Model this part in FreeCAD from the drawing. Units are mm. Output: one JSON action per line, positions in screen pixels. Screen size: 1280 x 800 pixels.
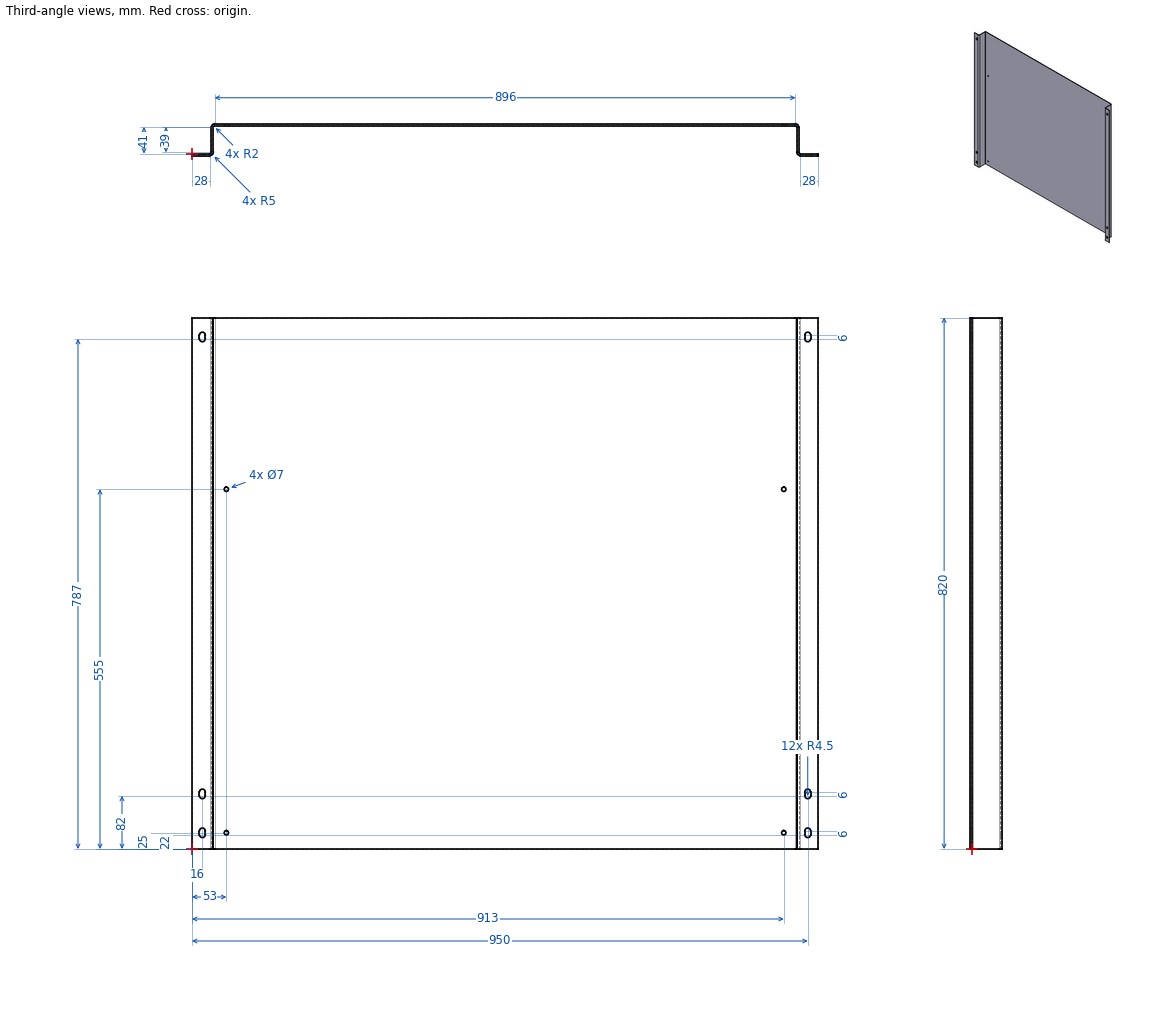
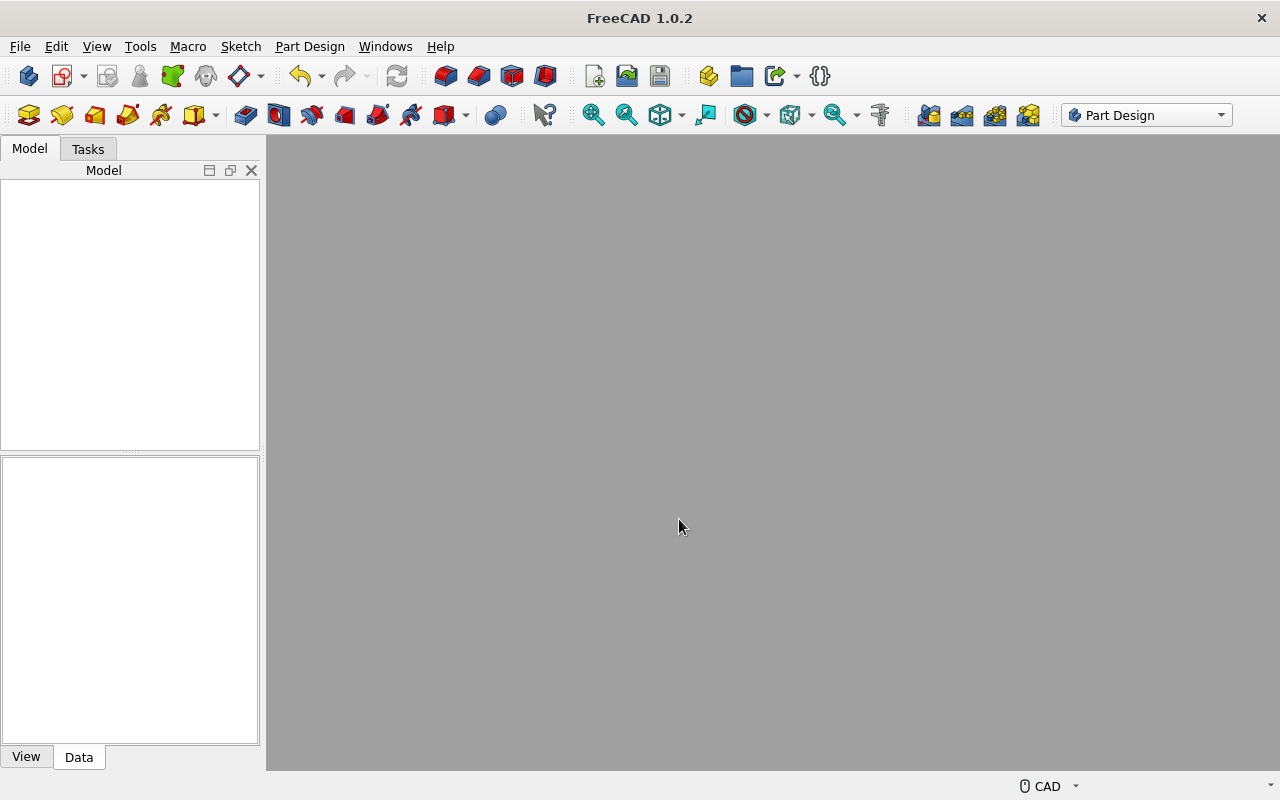
{"action": "key", "text": "ctrl+n"}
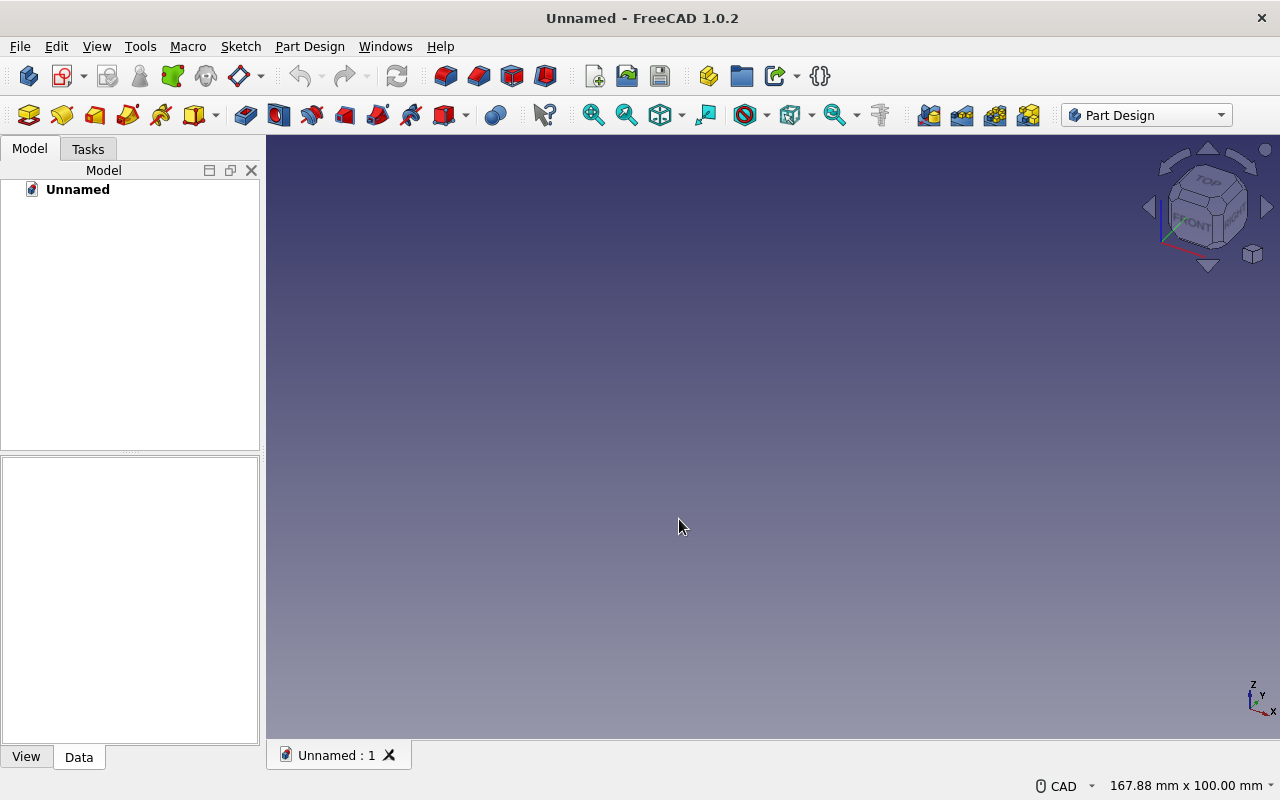
{"action": "left_click", "coordinate": [62, 76]}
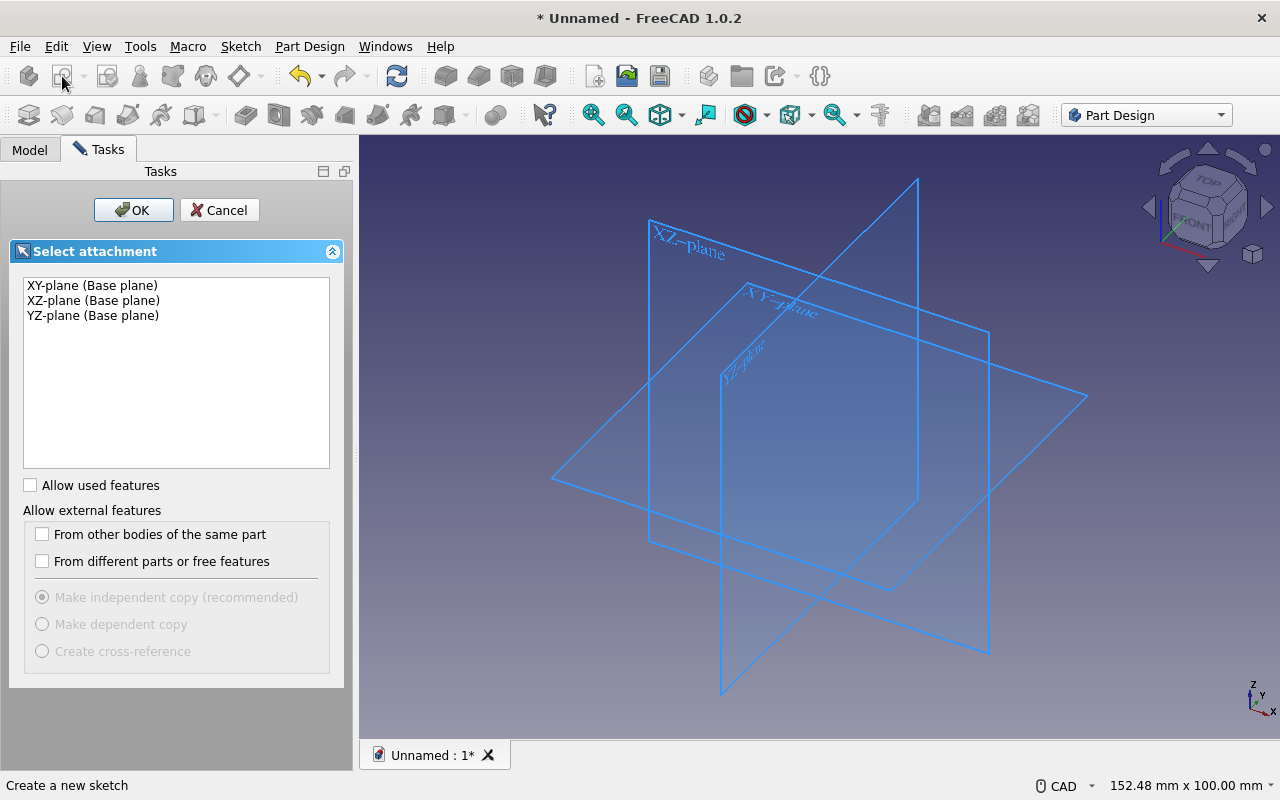
{"action": "left_click", "coordinate": [84, 286]}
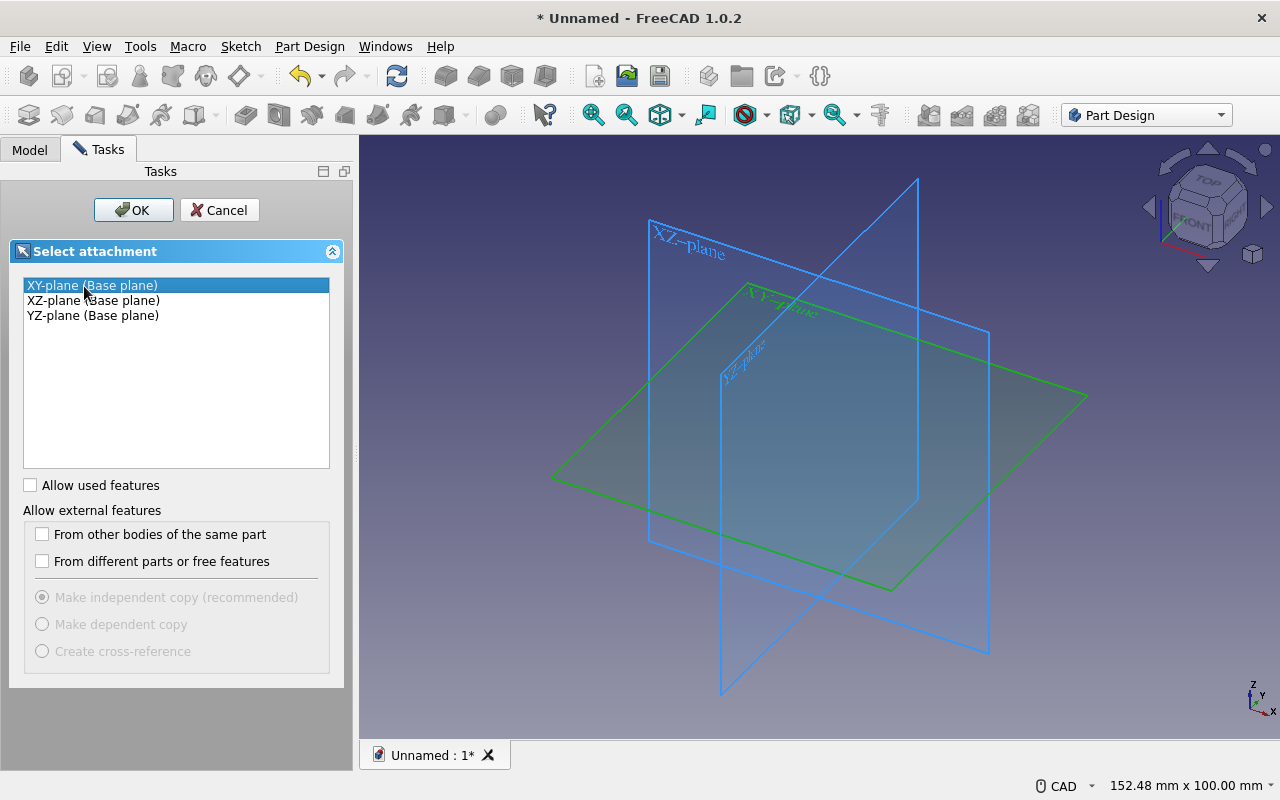
{"action": "left_click", "coordinate": [134, 210]}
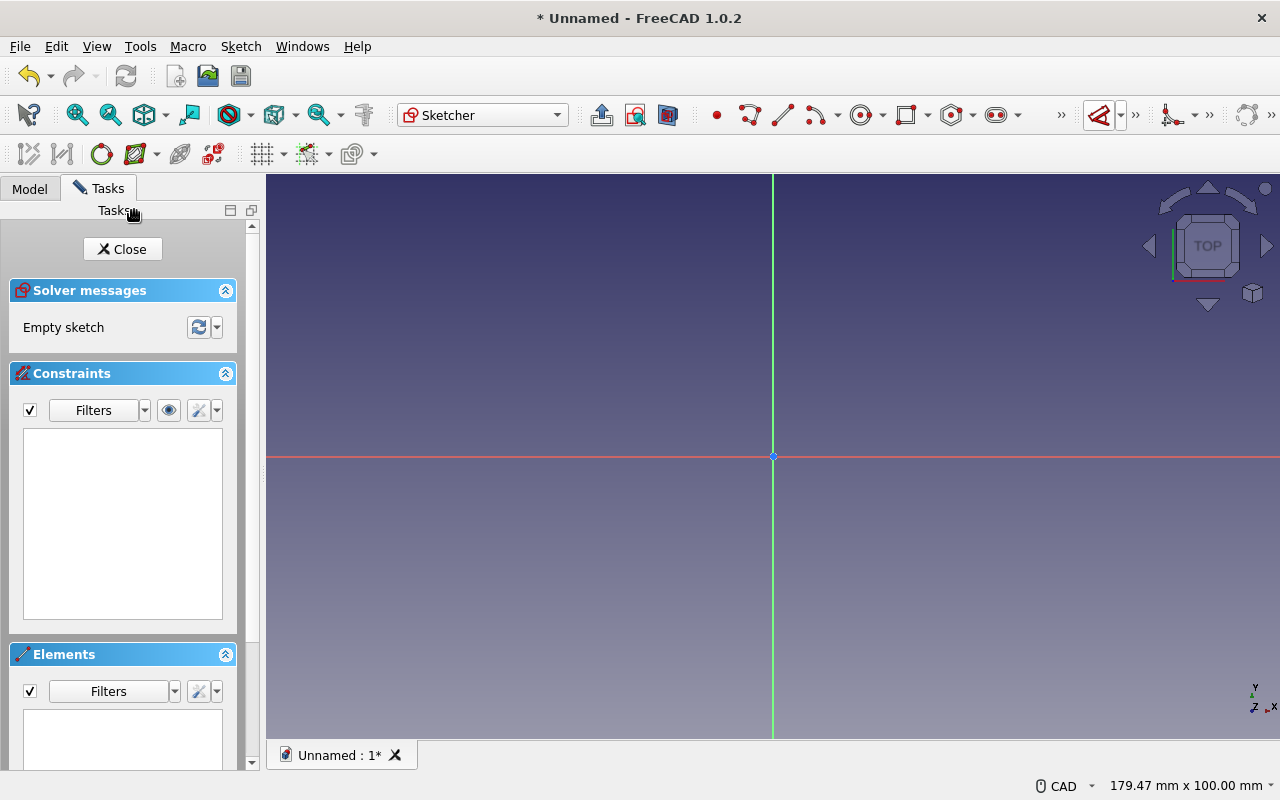
{"action": "scroll", "coordinate": [356, 472], "scroll_direction": "down", "scroll_amount": 11}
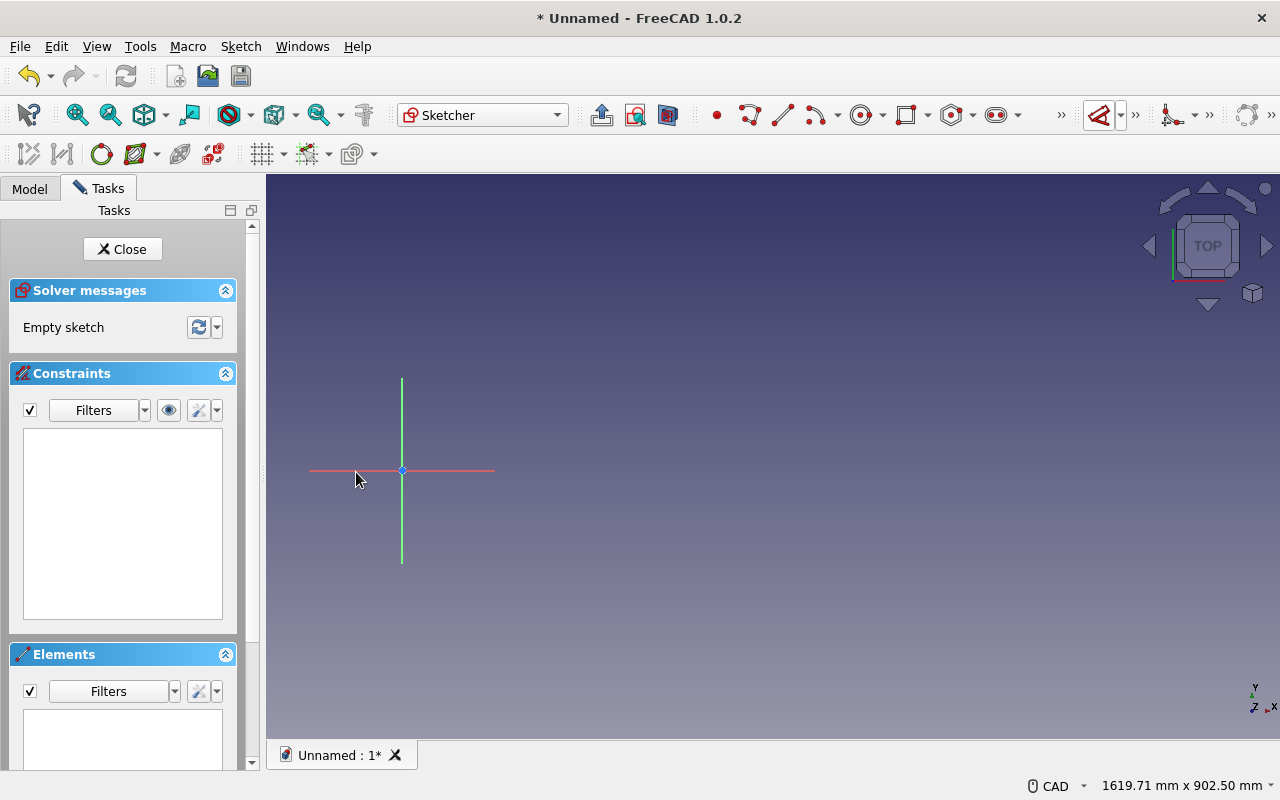
{"action": "left_click", "coordinate": [750, 116]}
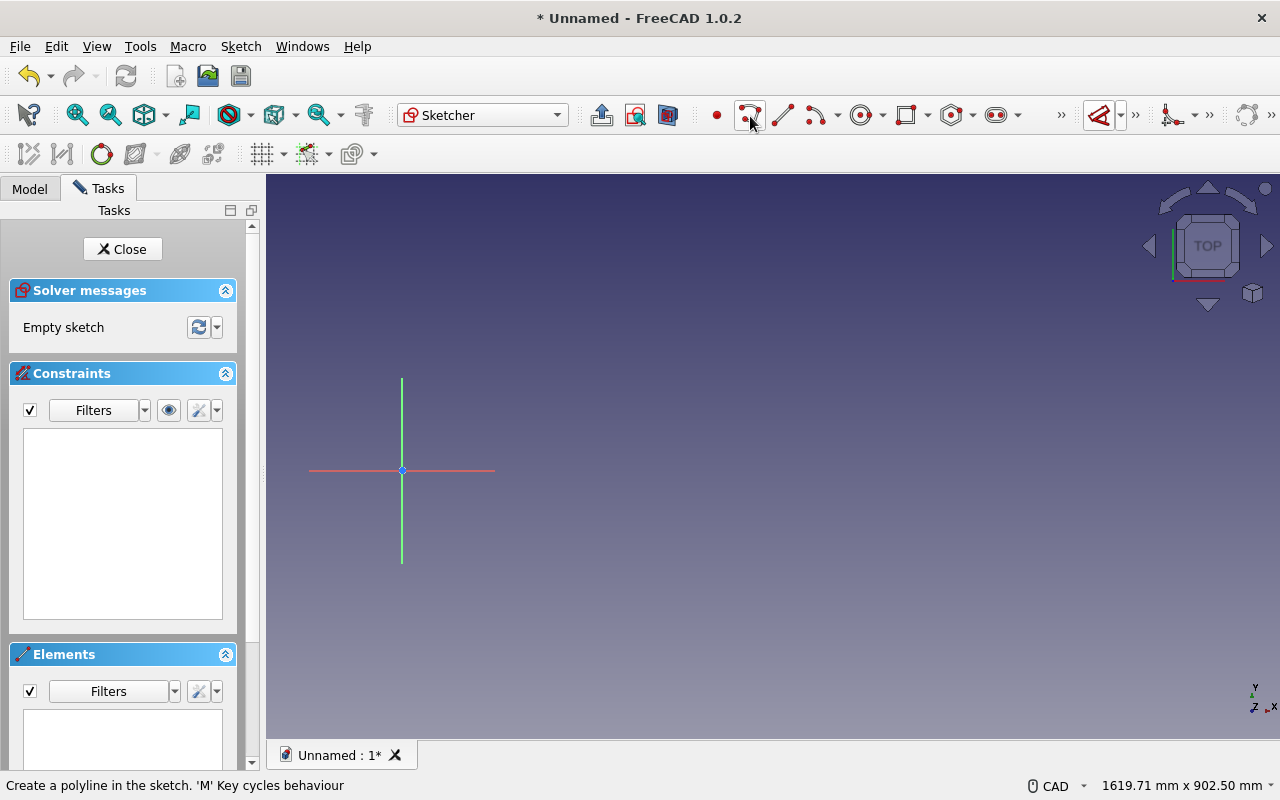
{"action": "left_click", "coordinate": [420, 471]}
{"action": "left_click", "coordinate": [402, 471]}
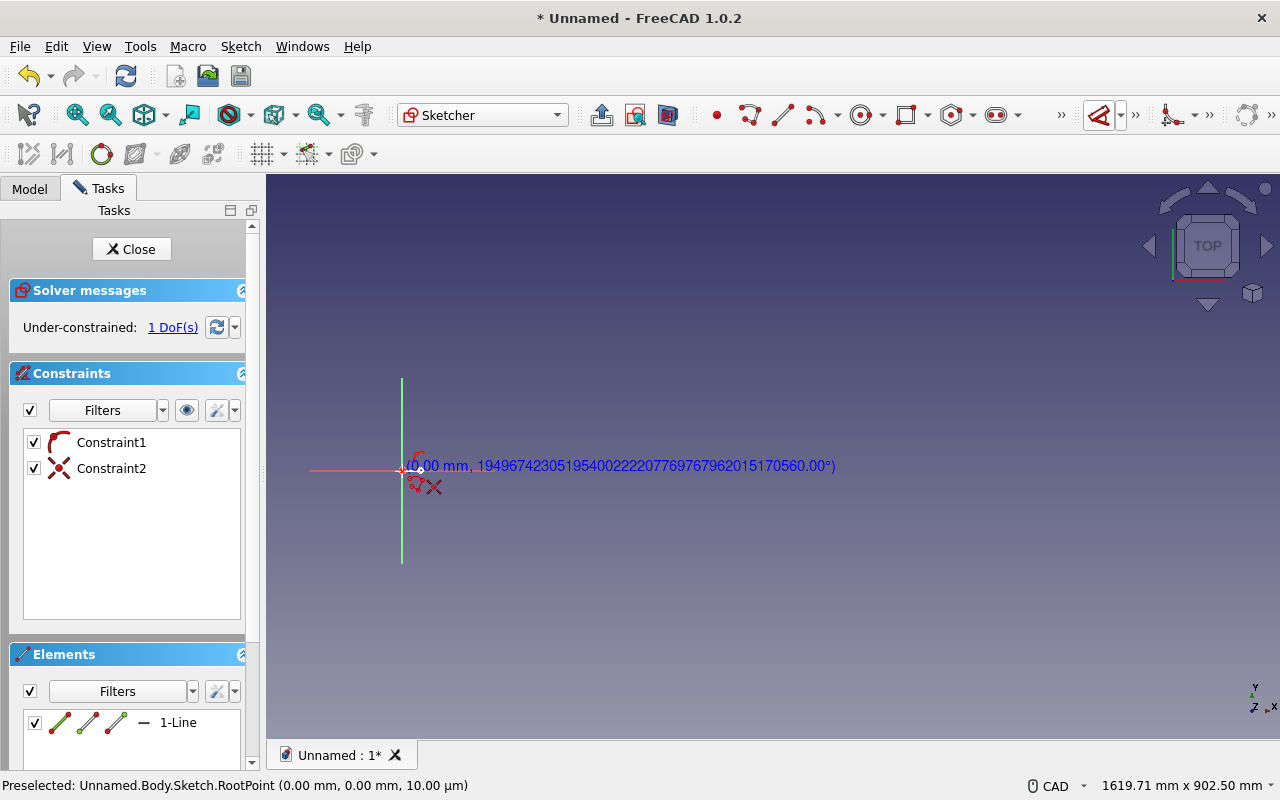
{"action": "scroll", "coordinate": [402, 473], "scroll_direction": "up", "scroll_amount": 11}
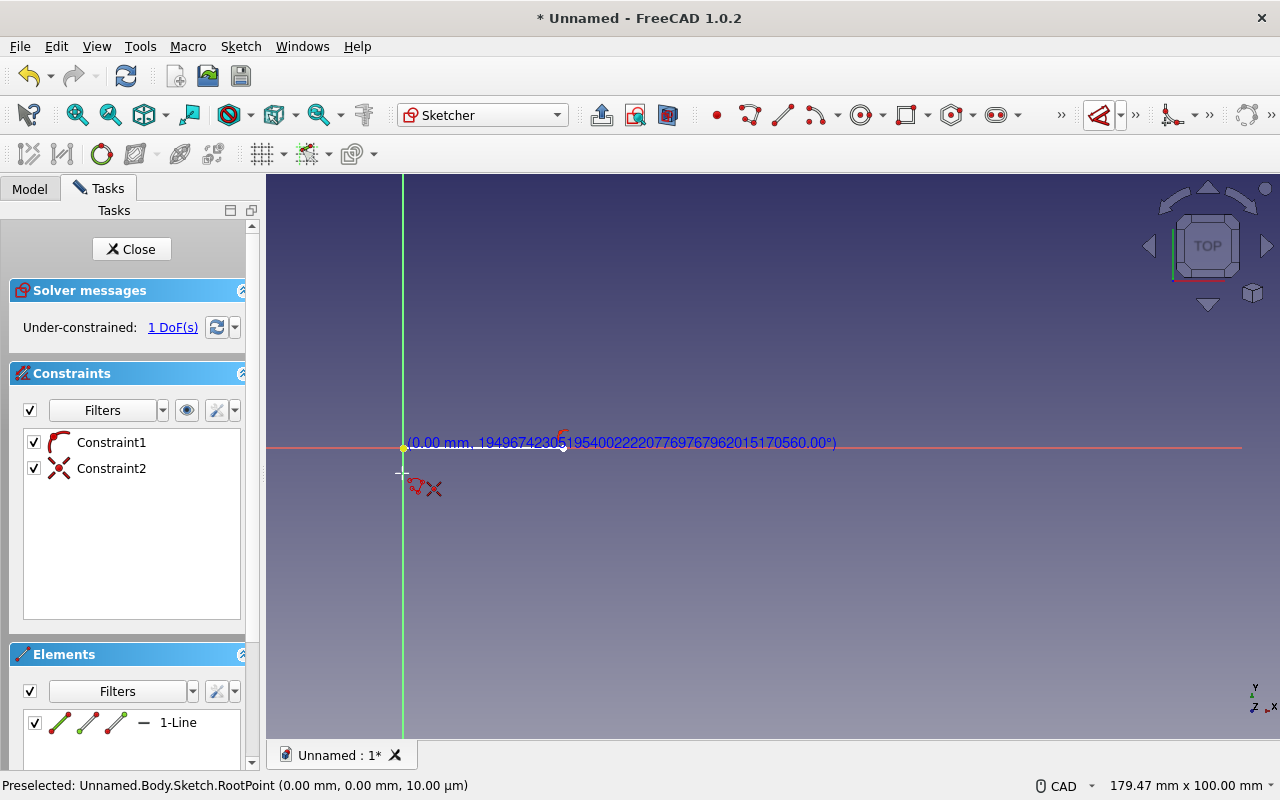
{"action": "left_click", "coordinate": [412, 465]}
{"action": "left_click", "coordinate": [562, 465]}
{"action": "right_click", "coordinate": [562, 465]}